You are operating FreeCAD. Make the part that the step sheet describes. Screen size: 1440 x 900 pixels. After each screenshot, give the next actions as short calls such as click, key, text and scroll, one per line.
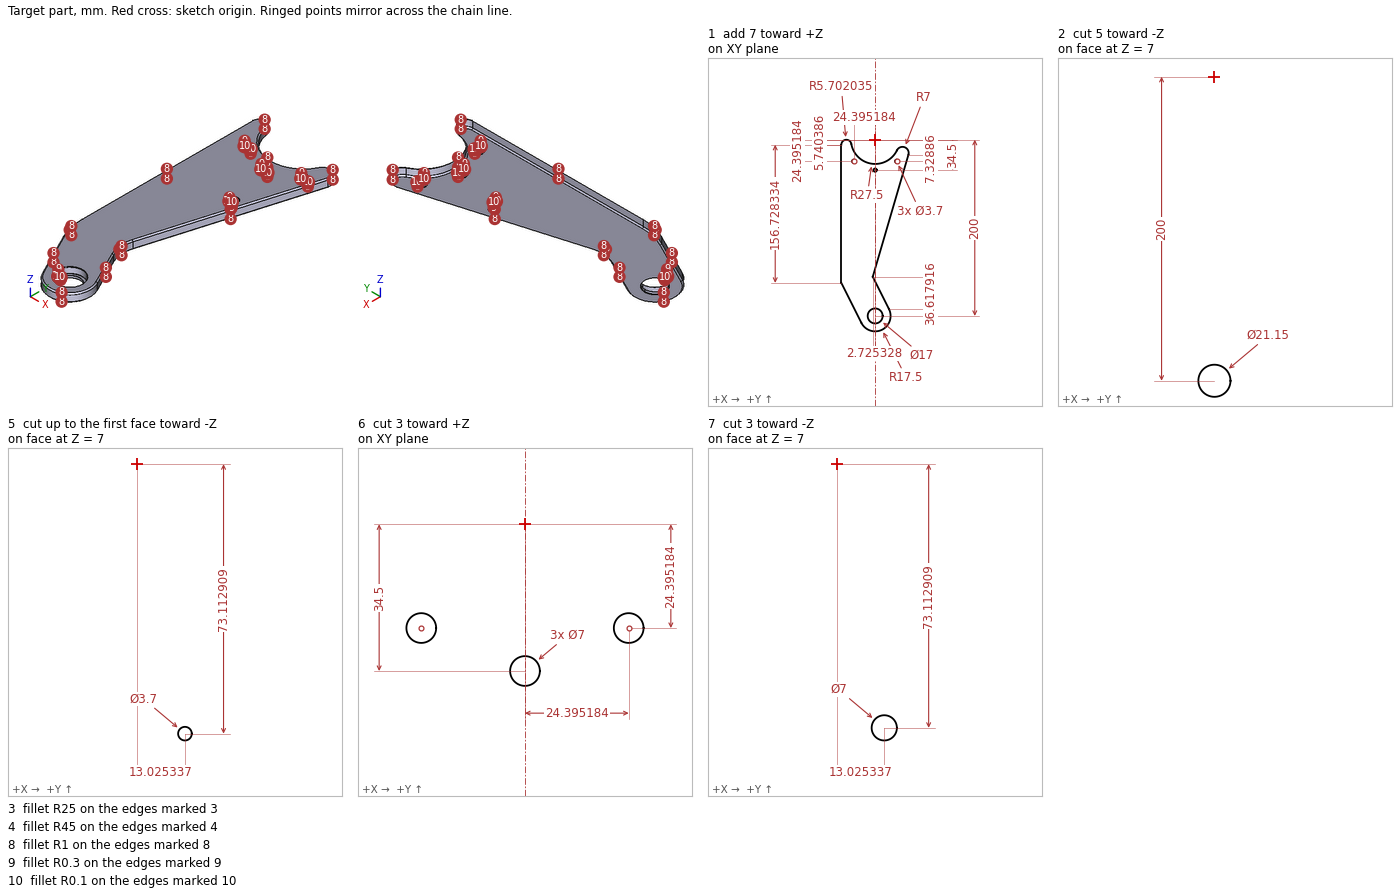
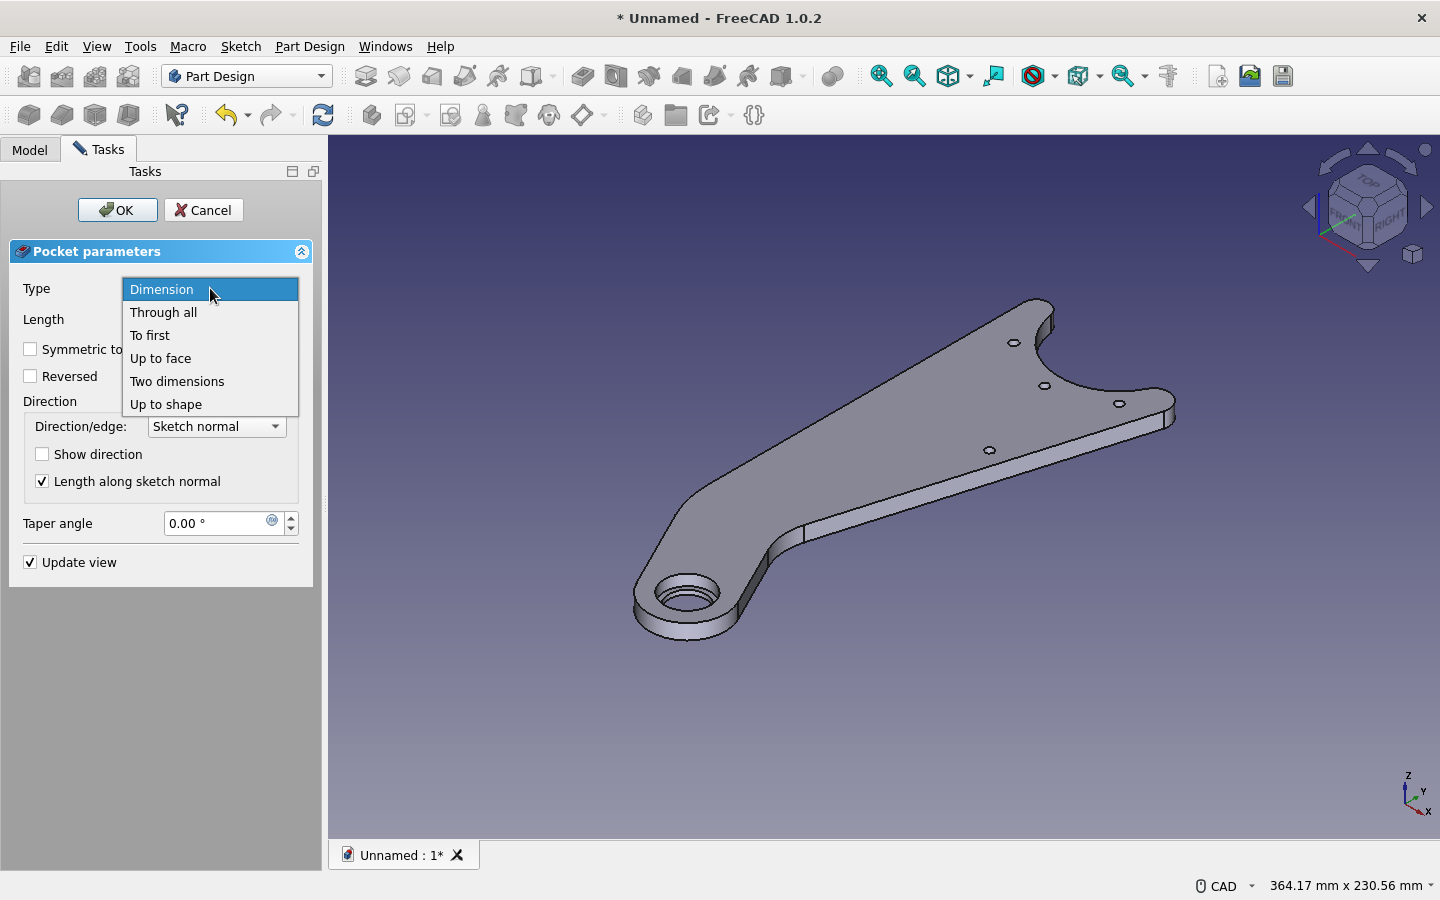
click(208, 336)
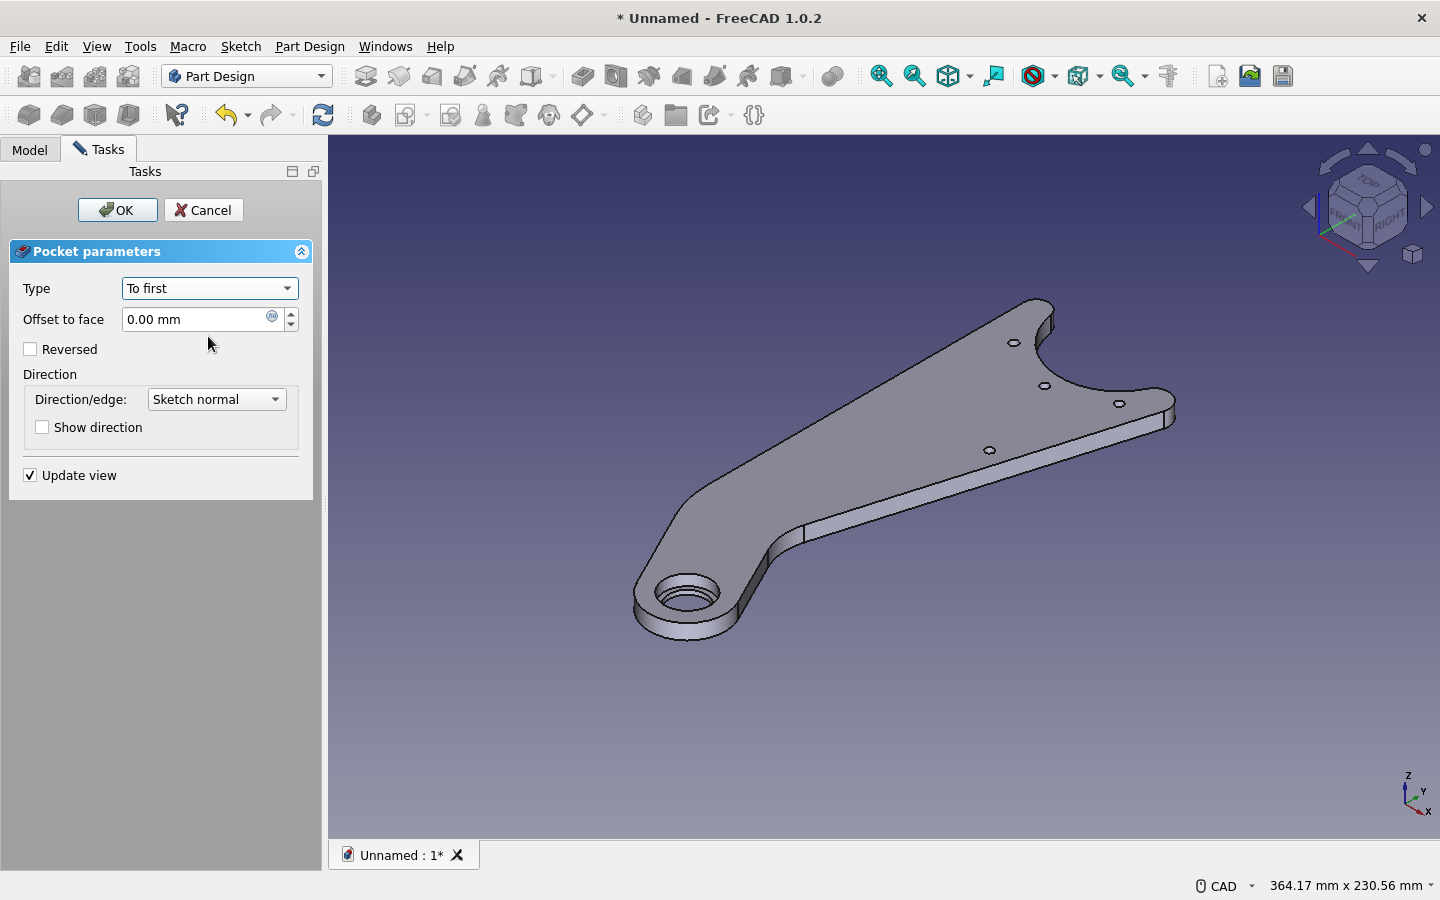
click(118, 210)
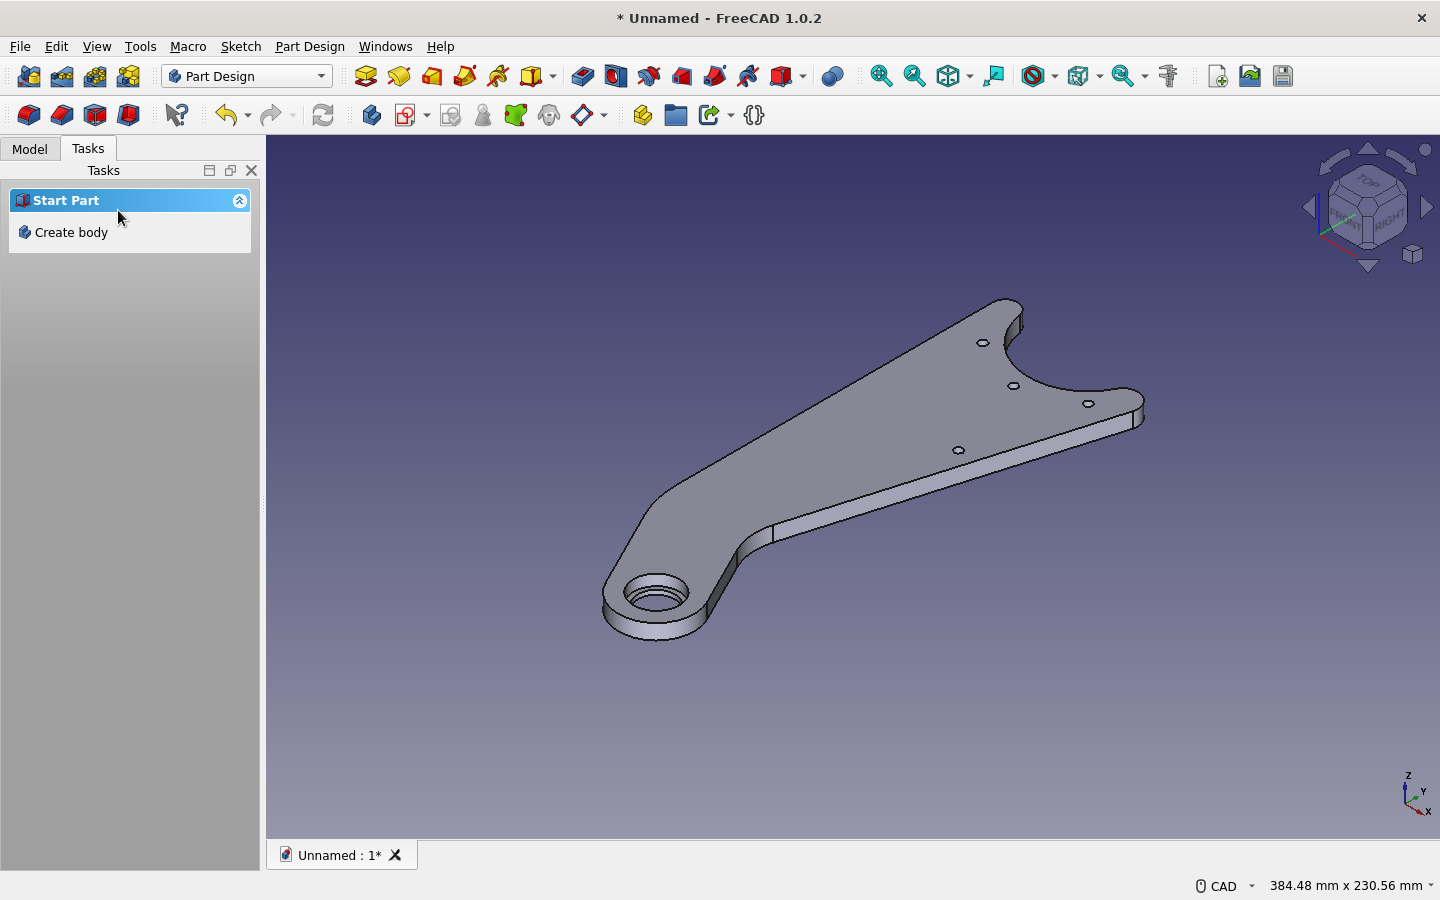
click(404, 116)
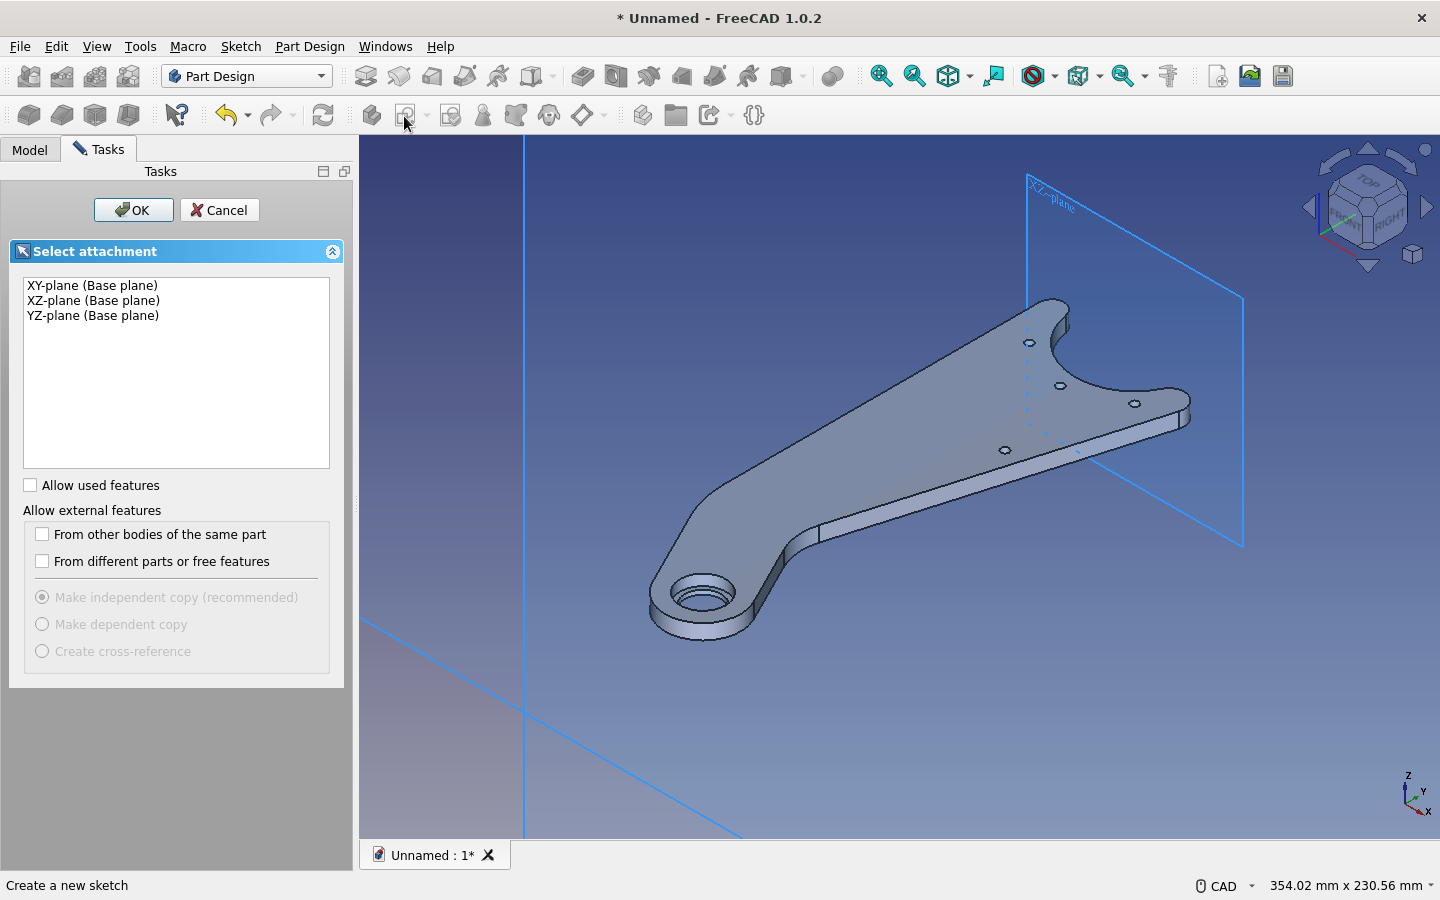
click(84, 286)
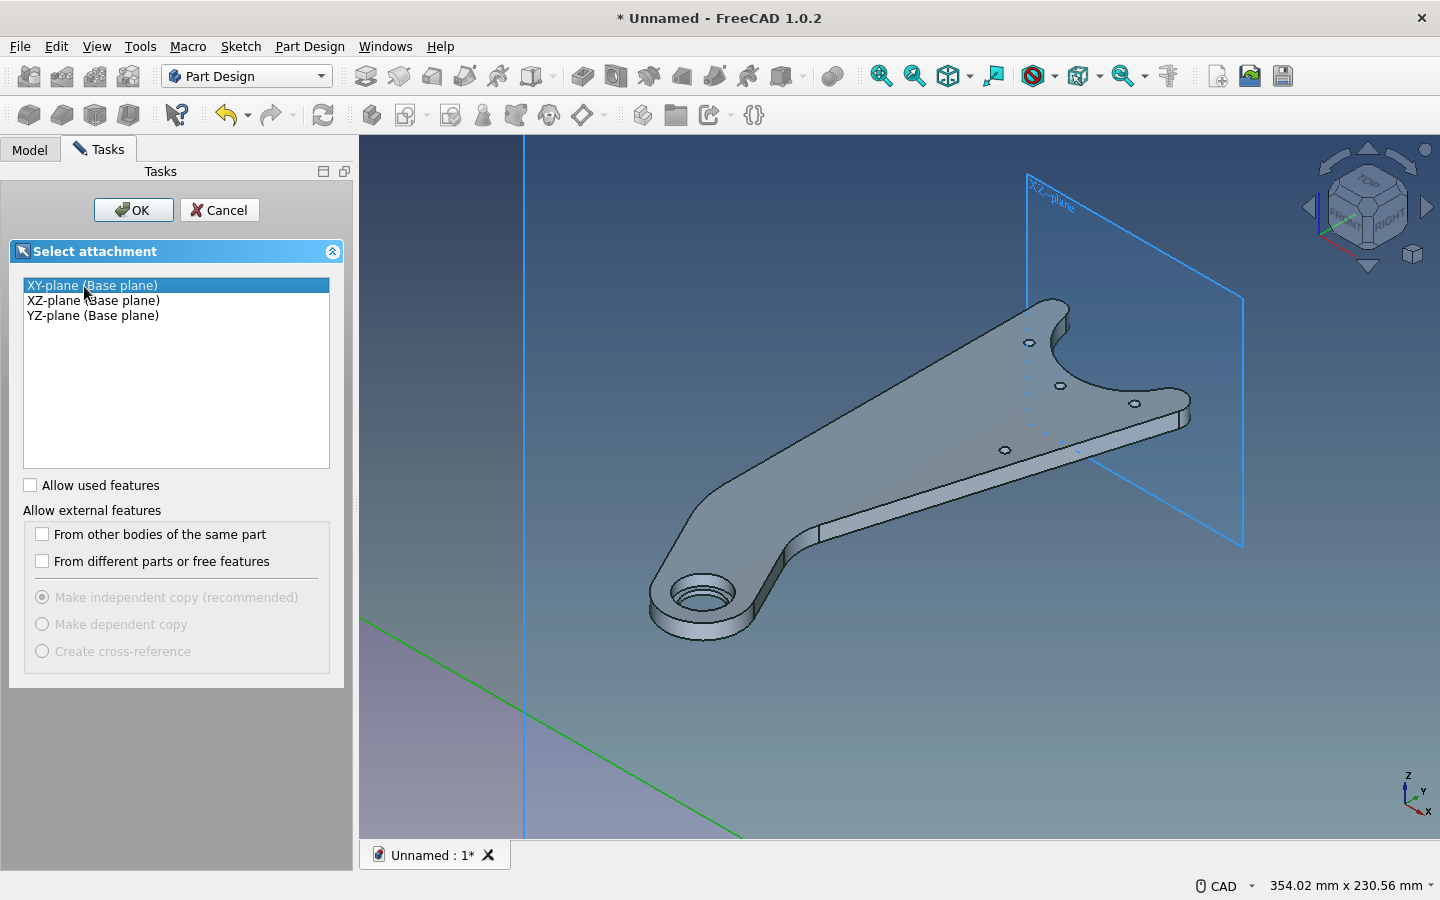
click(134, 210)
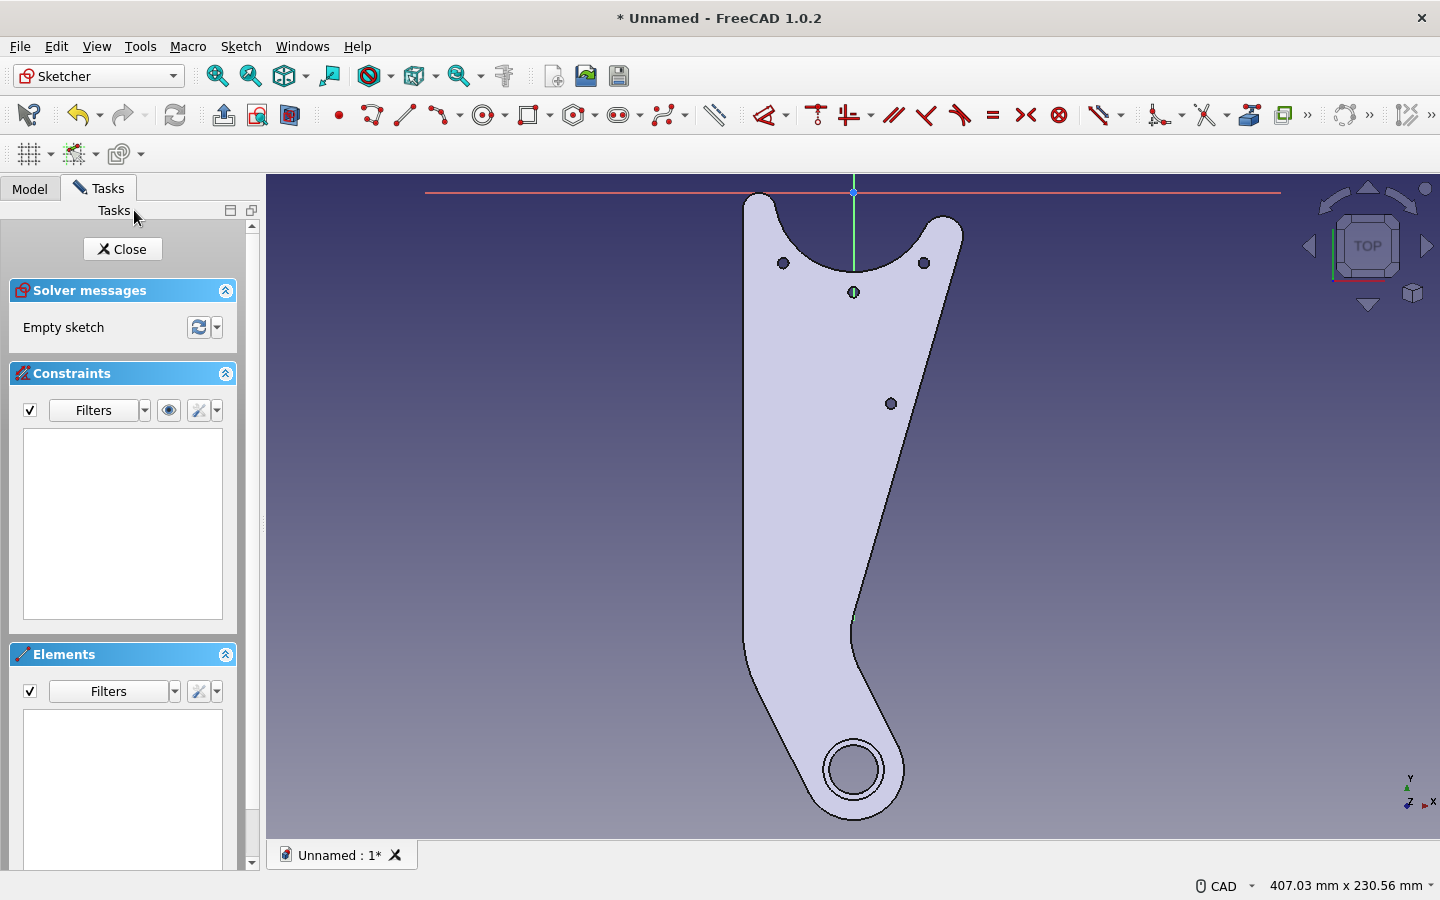
click(290, 116)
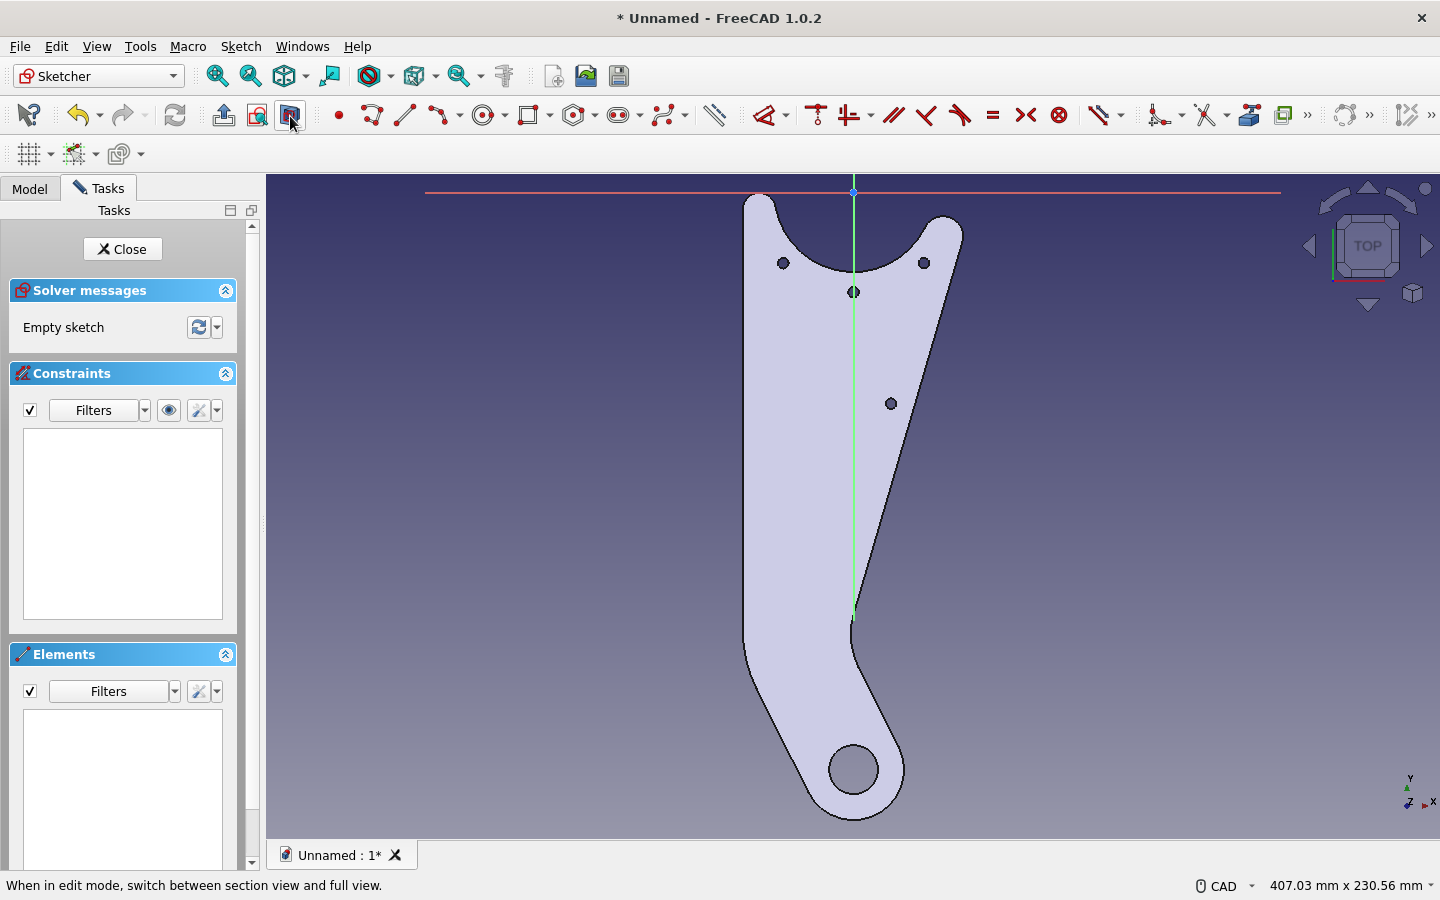
scroll(784, 506, down, 5)